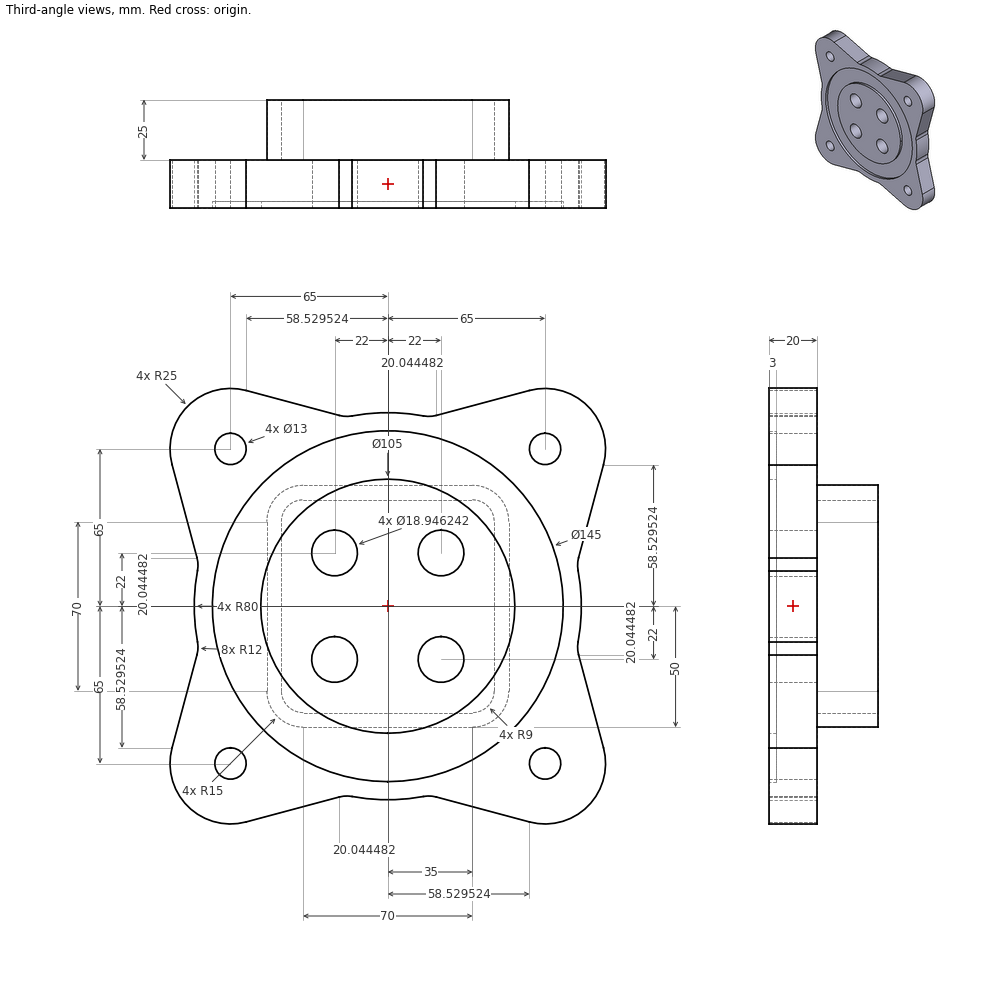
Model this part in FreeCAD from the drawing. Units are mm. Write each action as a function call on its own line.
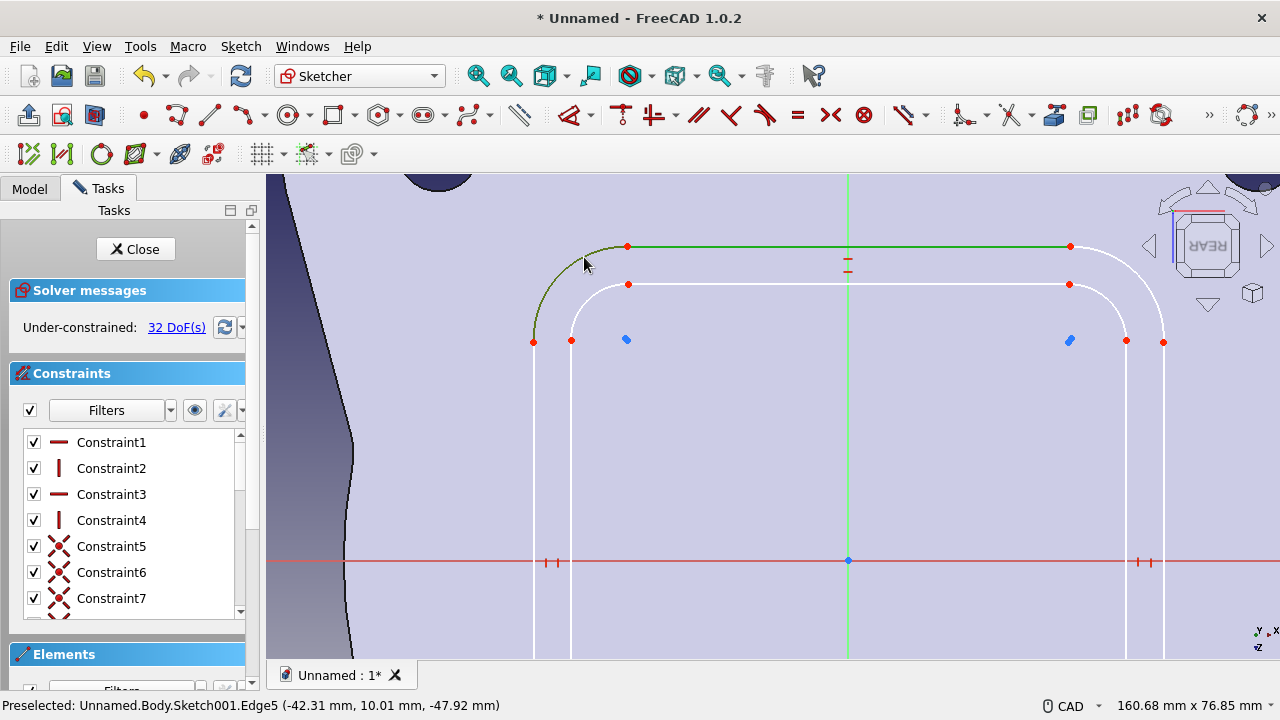
click(765, 116)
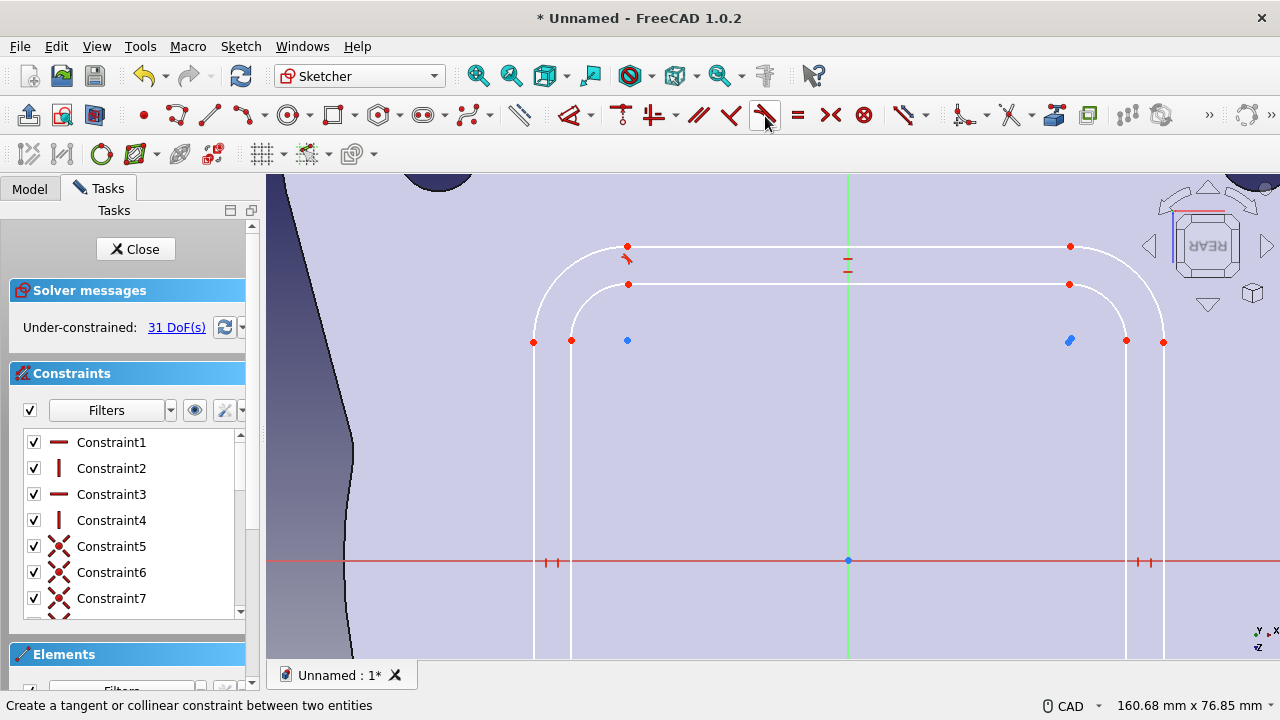
click(937, 247)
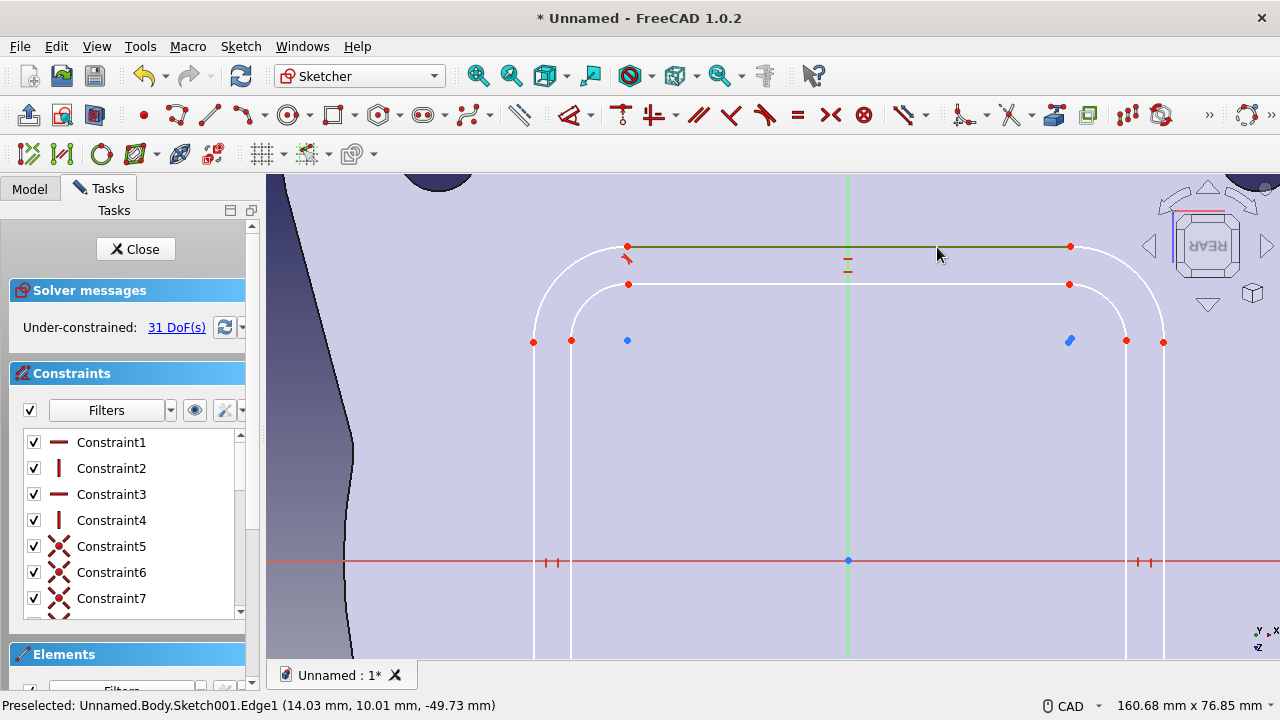
click(1114, 257)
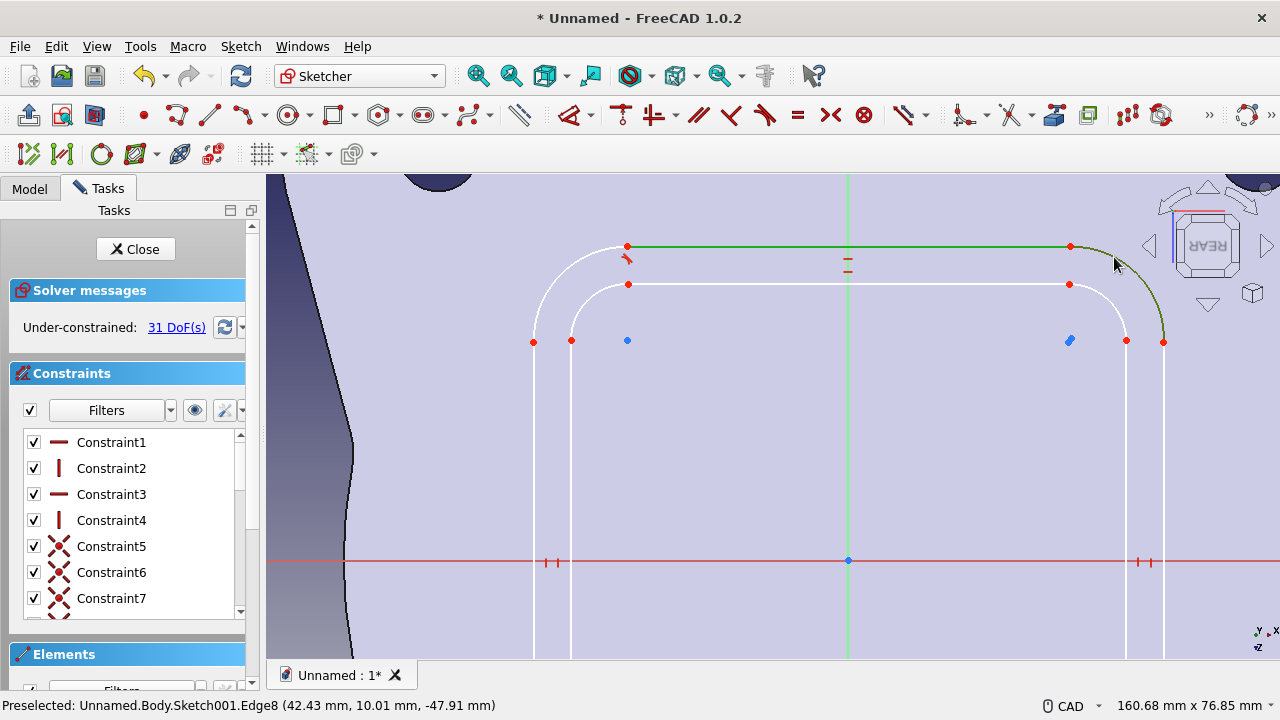
click(765, 116)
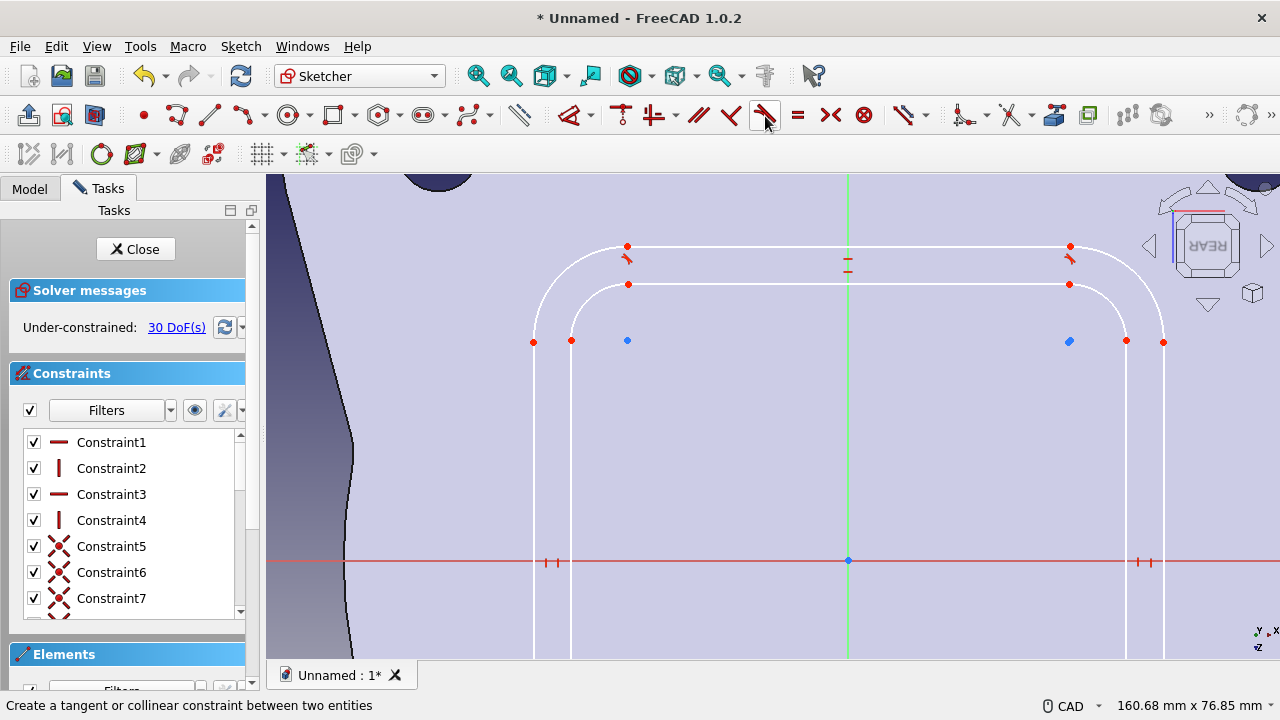
click(534, 475)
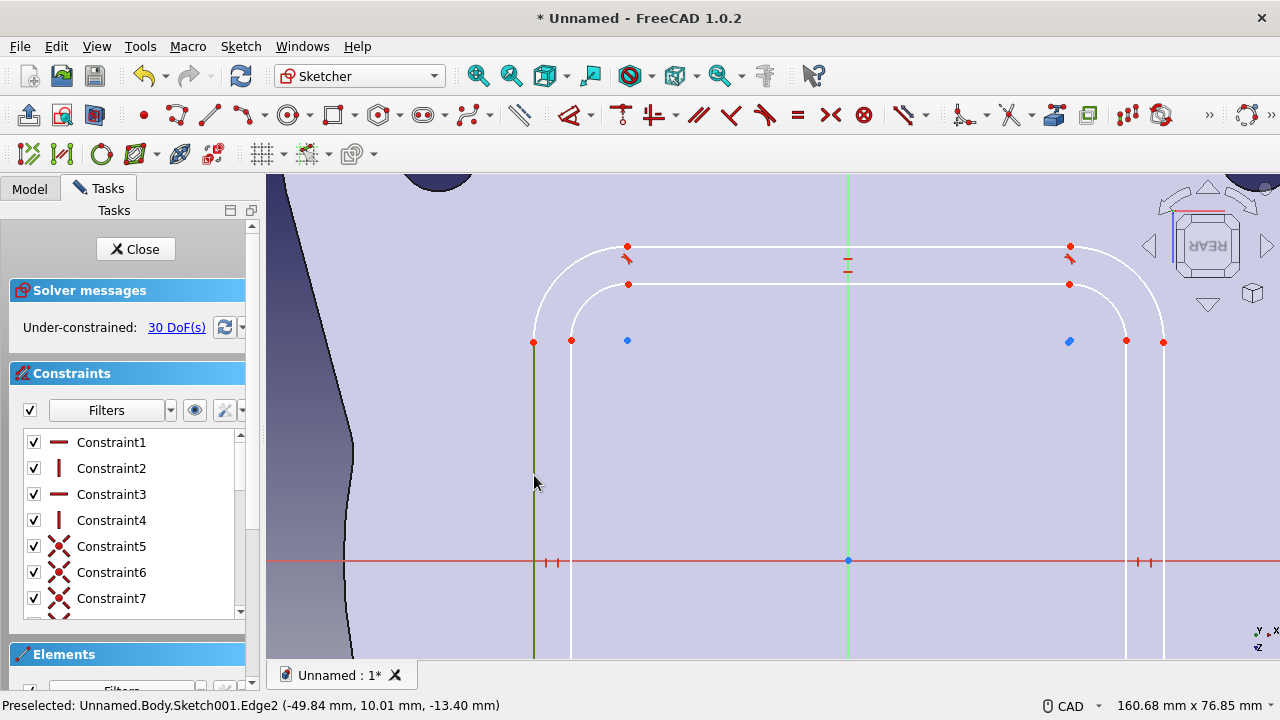
click(584, 257)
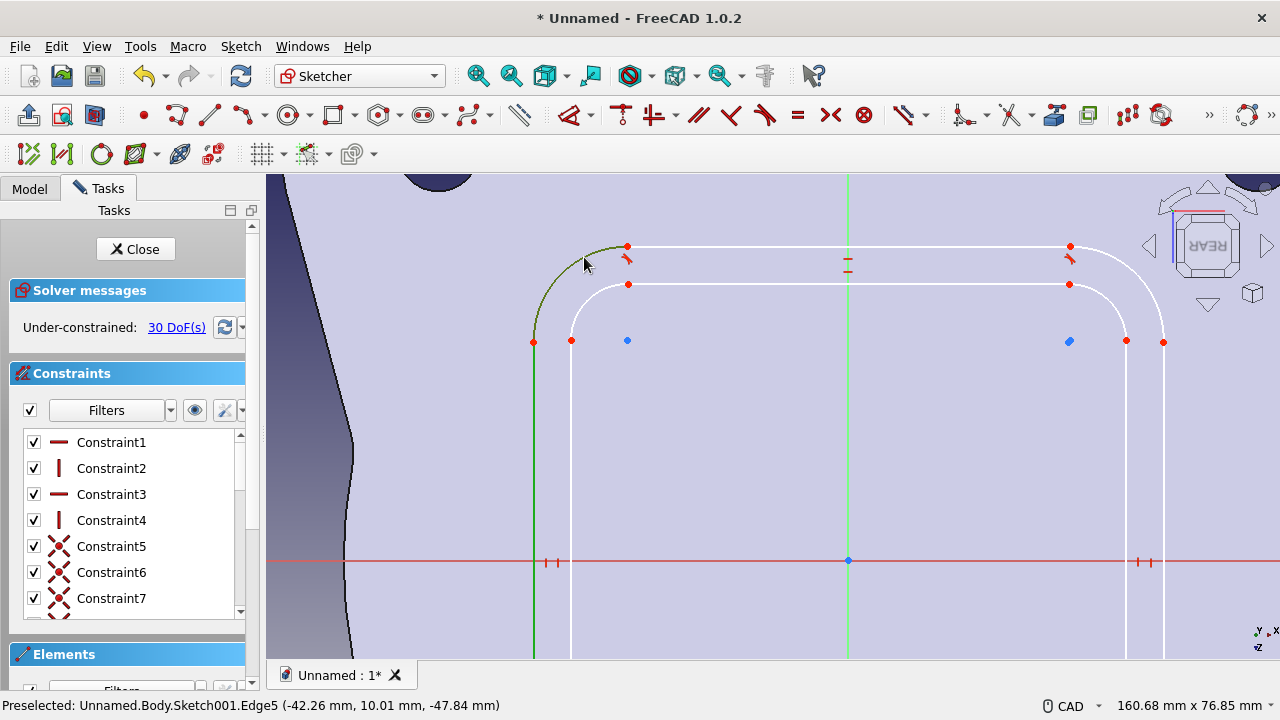
click(765, 116)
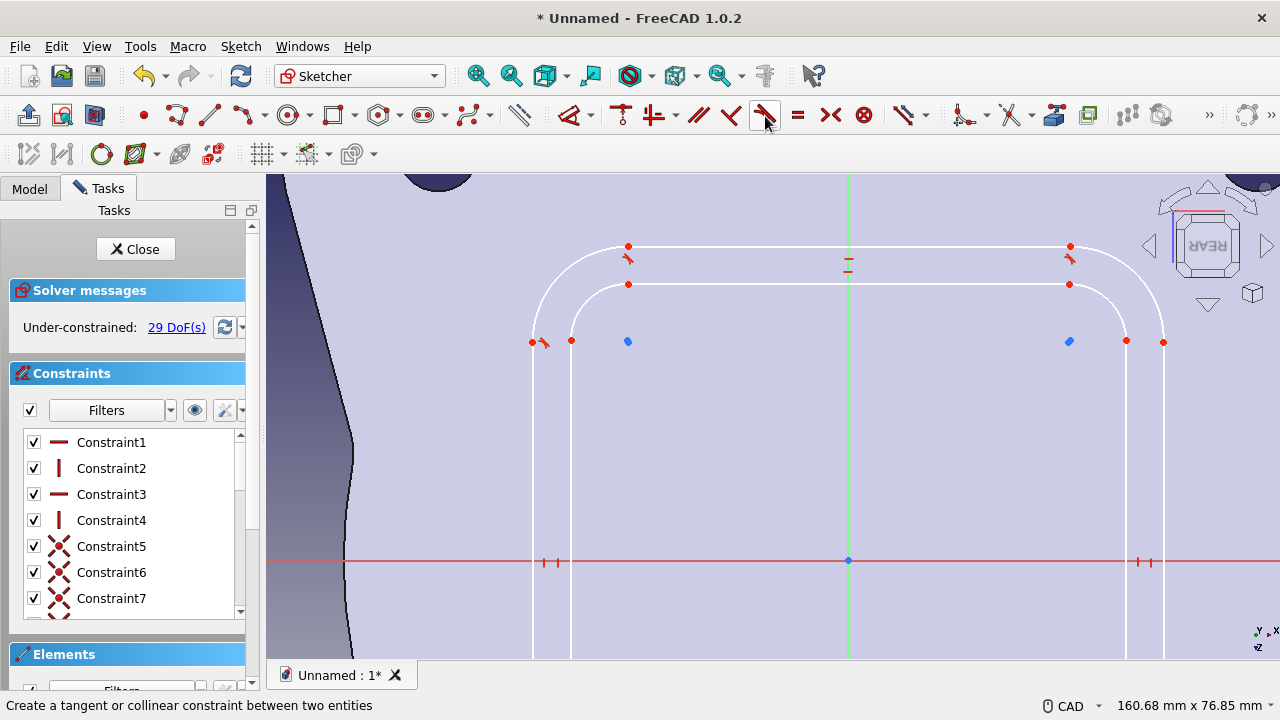
click(533, 475)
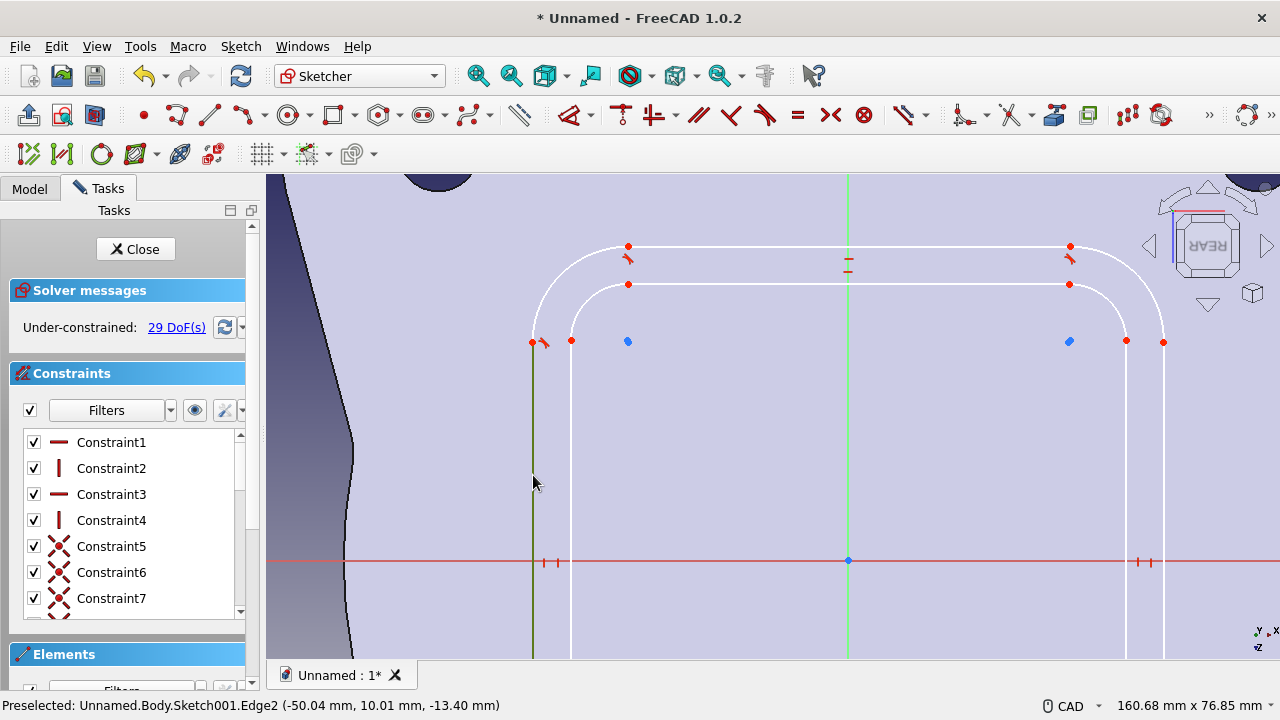
scroll(587, 299, down, 4)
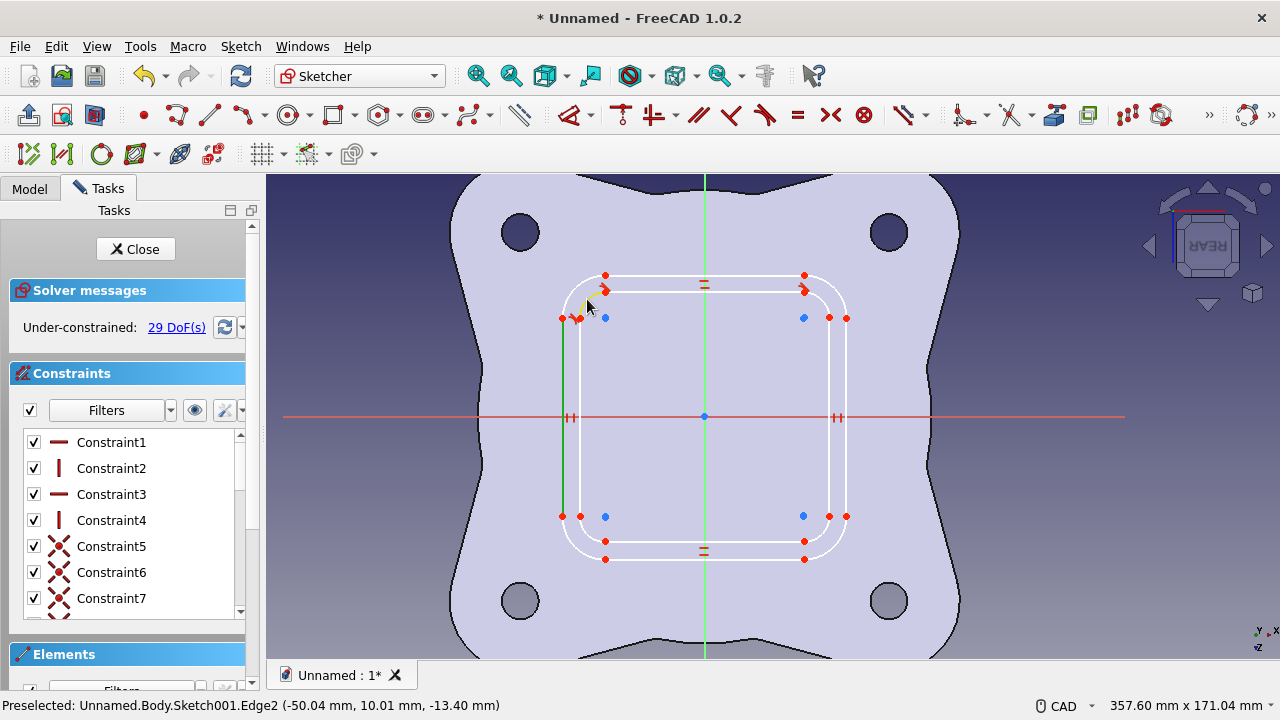
click(567, 536)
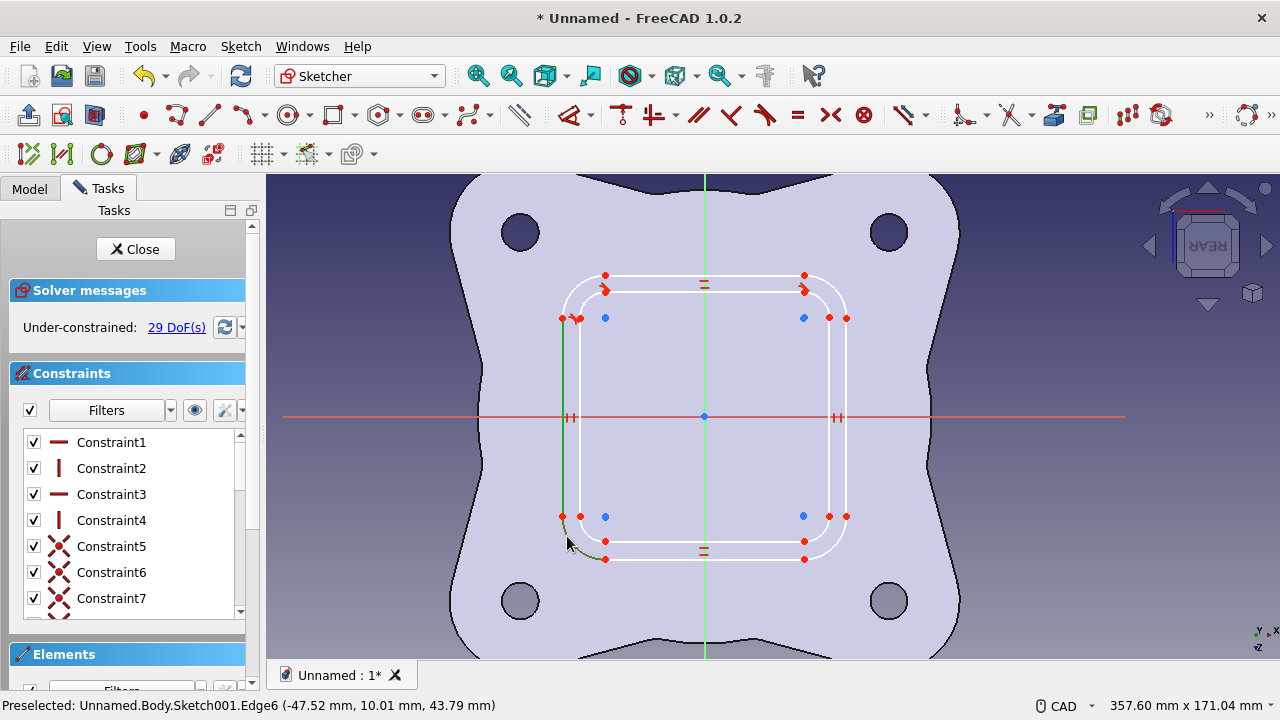
click(765, 116)